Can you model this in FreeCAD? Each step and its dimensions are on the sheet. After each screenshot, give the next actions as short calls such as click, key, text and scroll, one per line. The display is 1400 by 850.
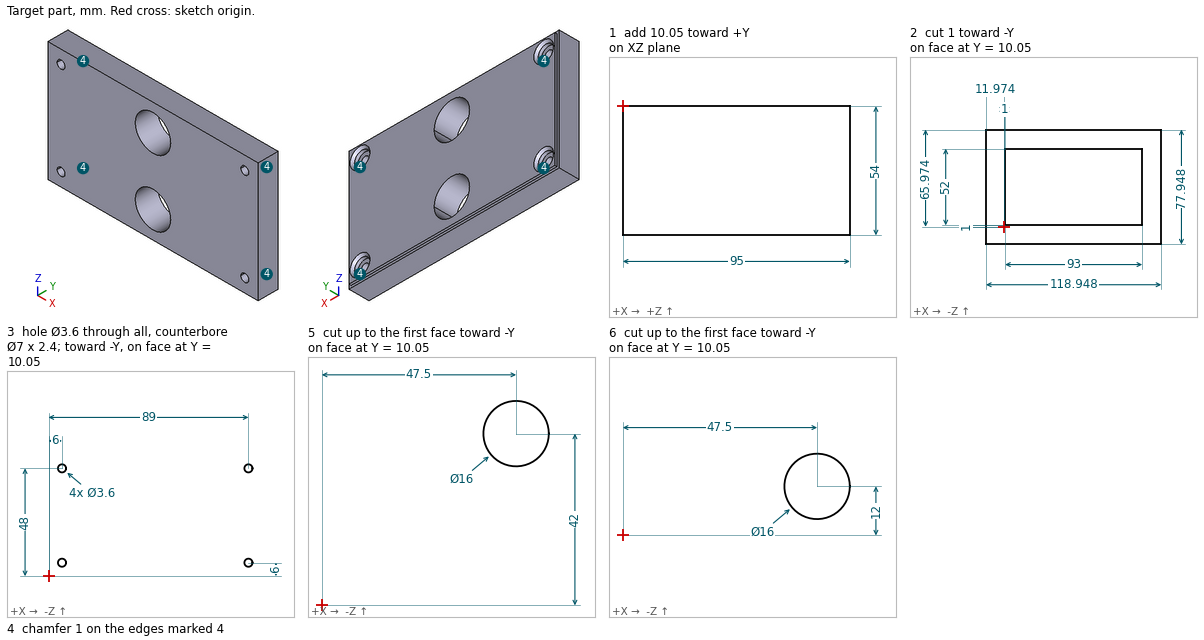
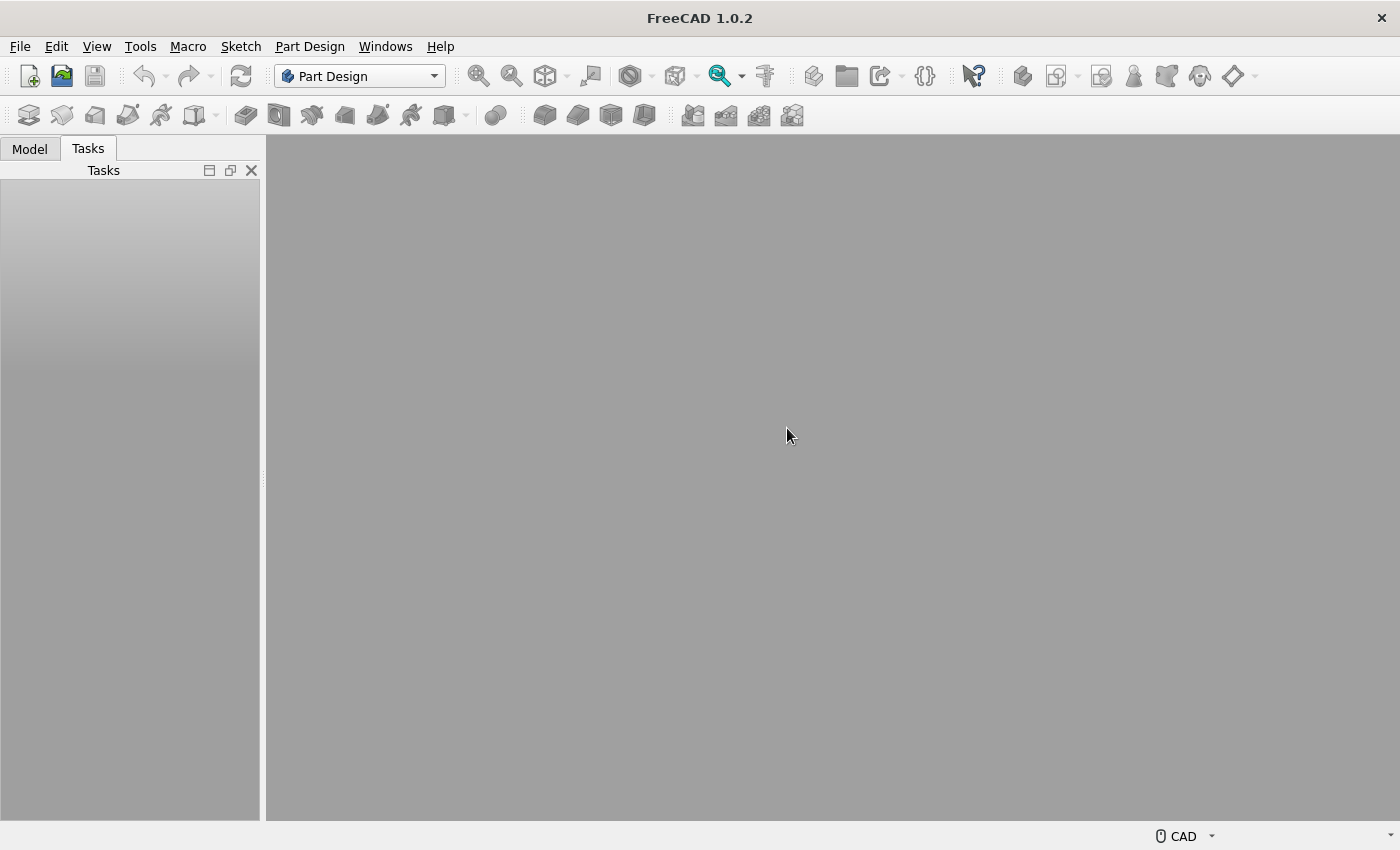
click(29, 76)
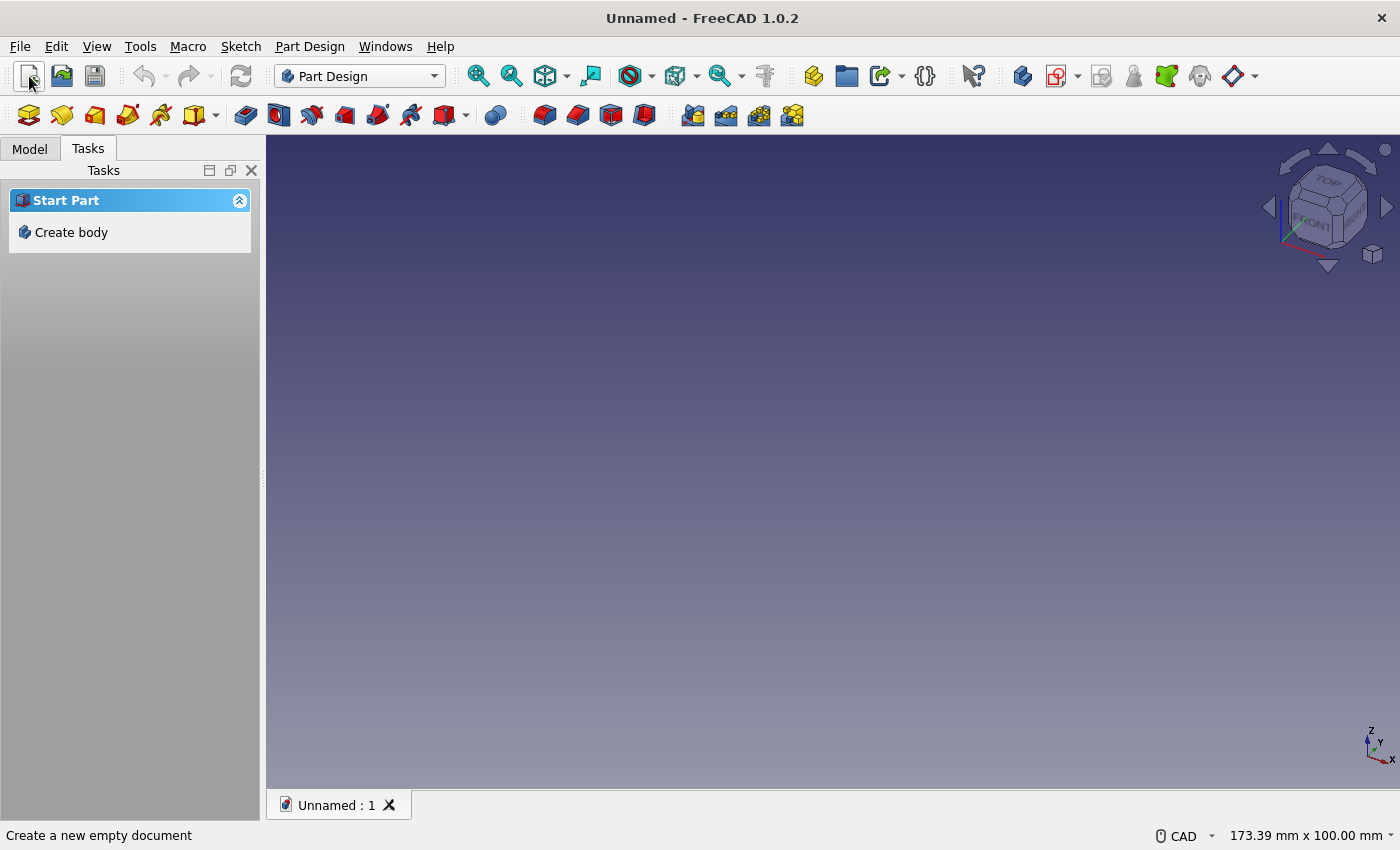
click(1056, 76)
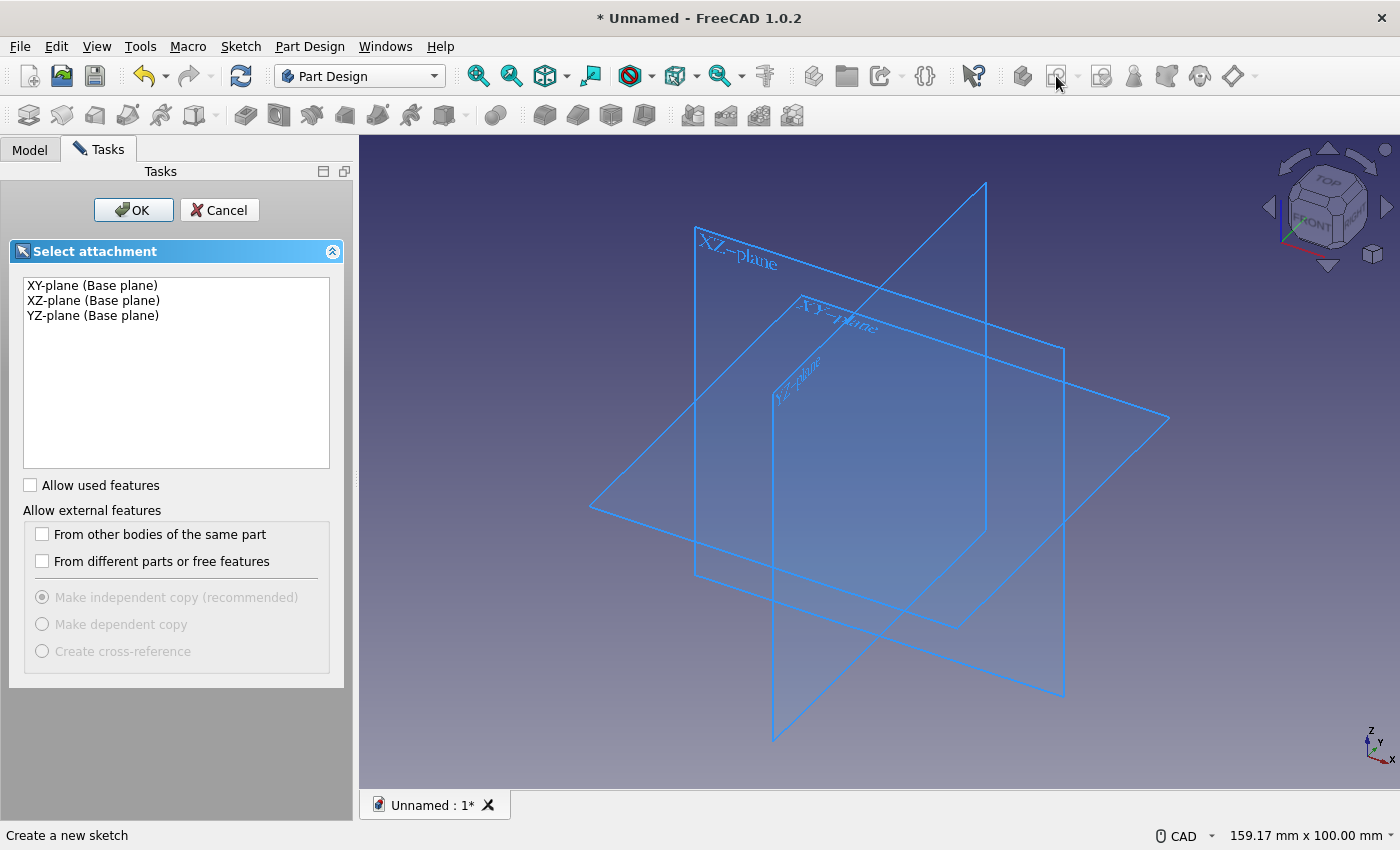
click(84, 300)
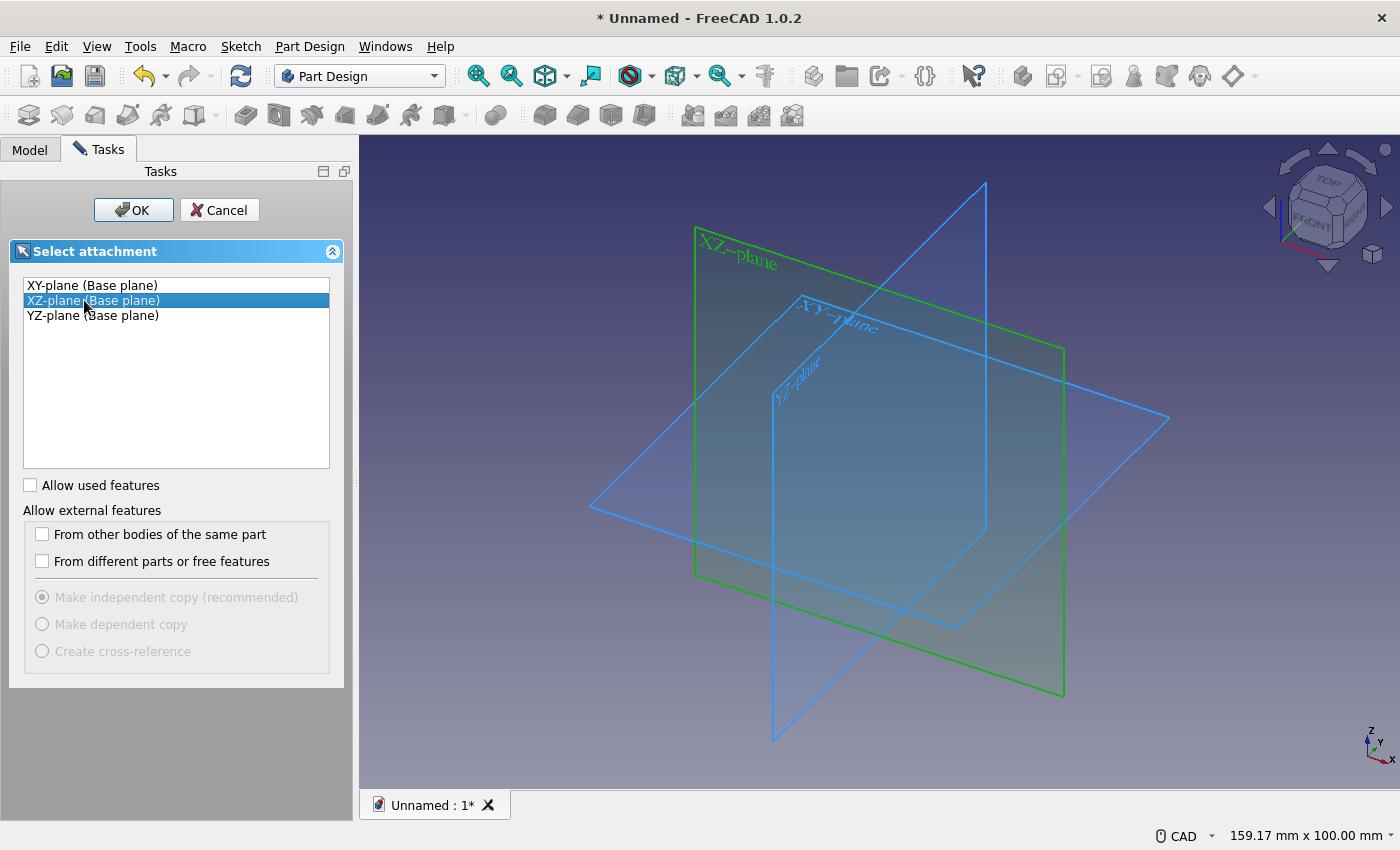
click(134, 210)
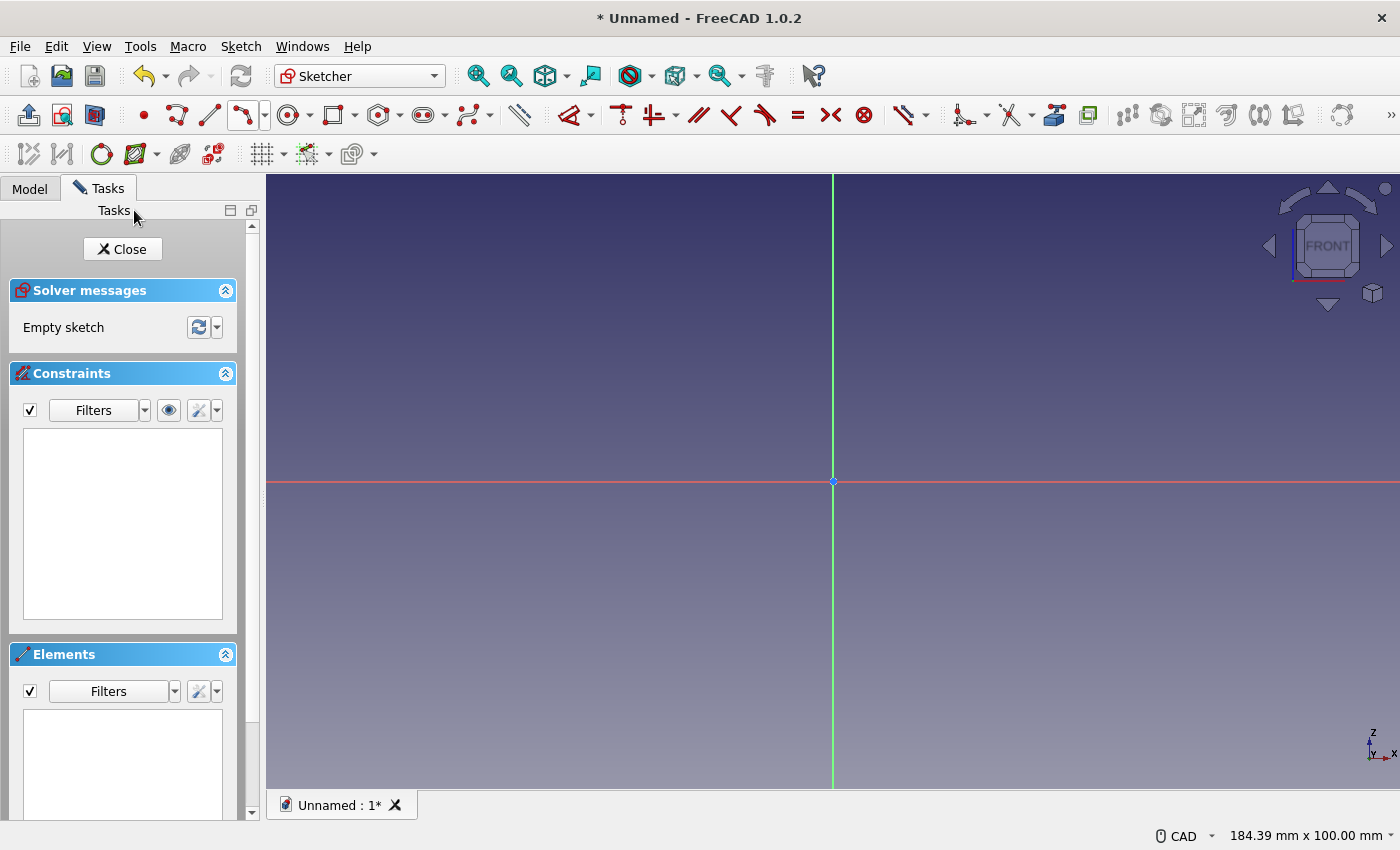
scroll(294, 202, down, 2)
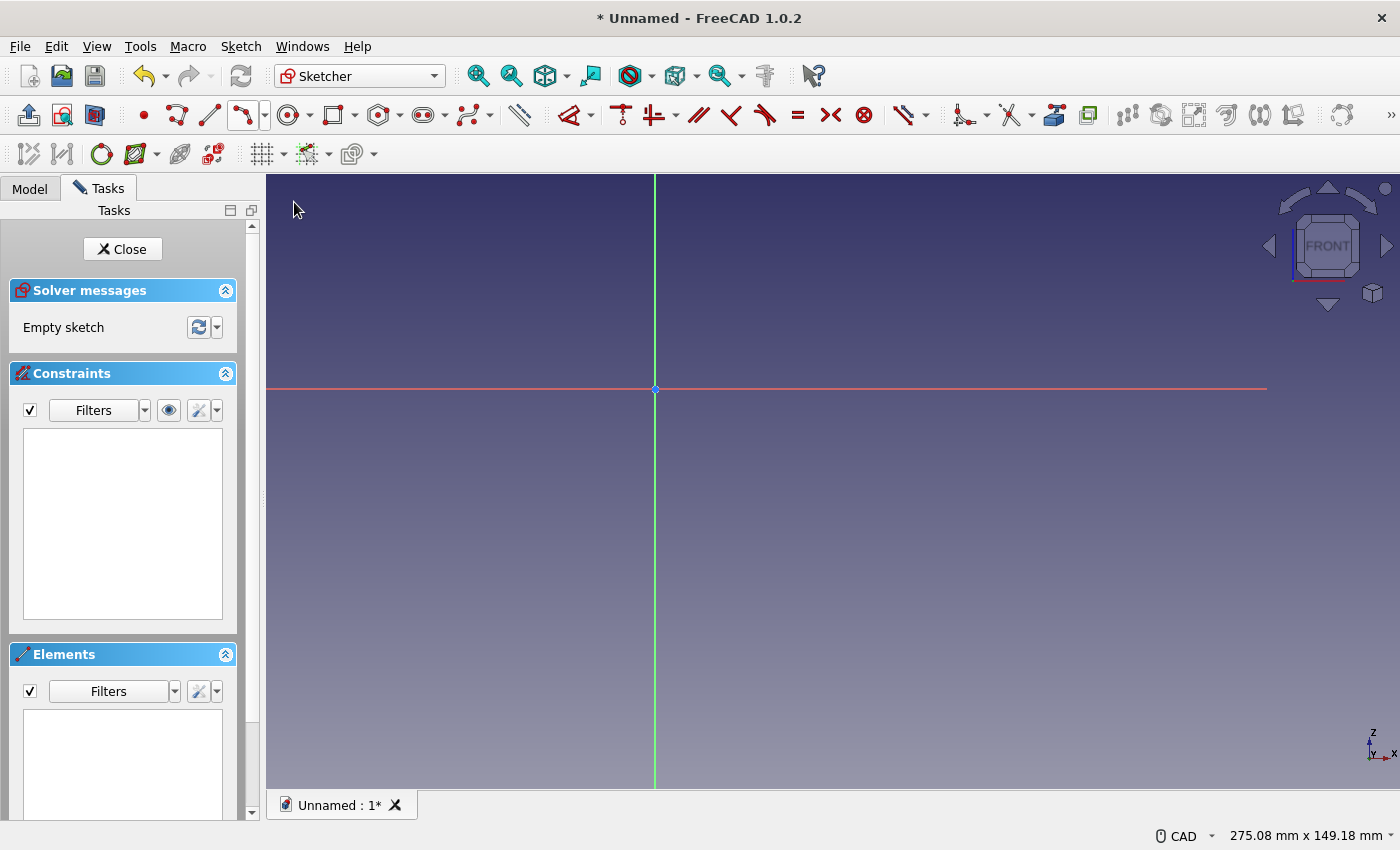
scroll(956, 524, up, 3)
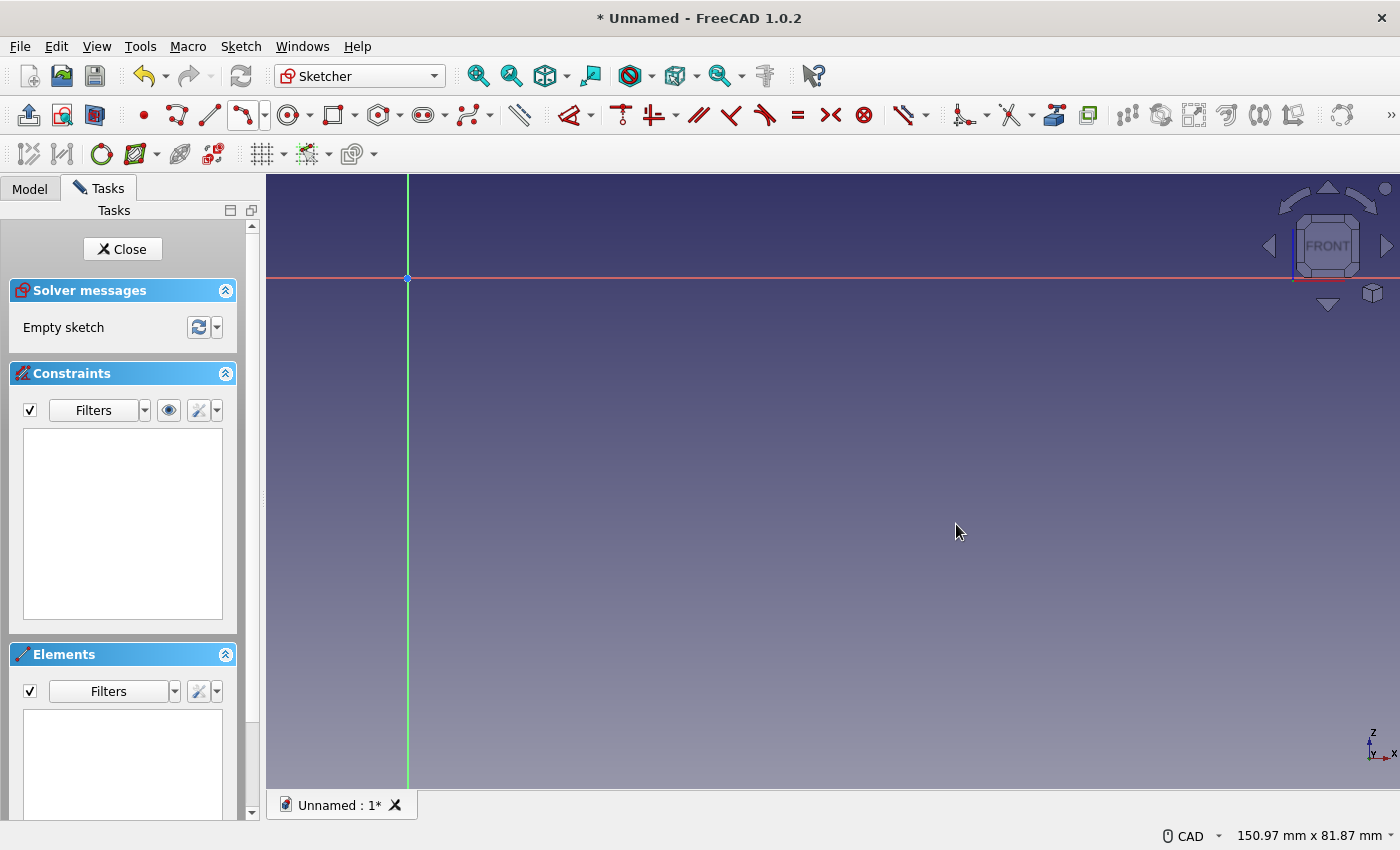
click(332, 116)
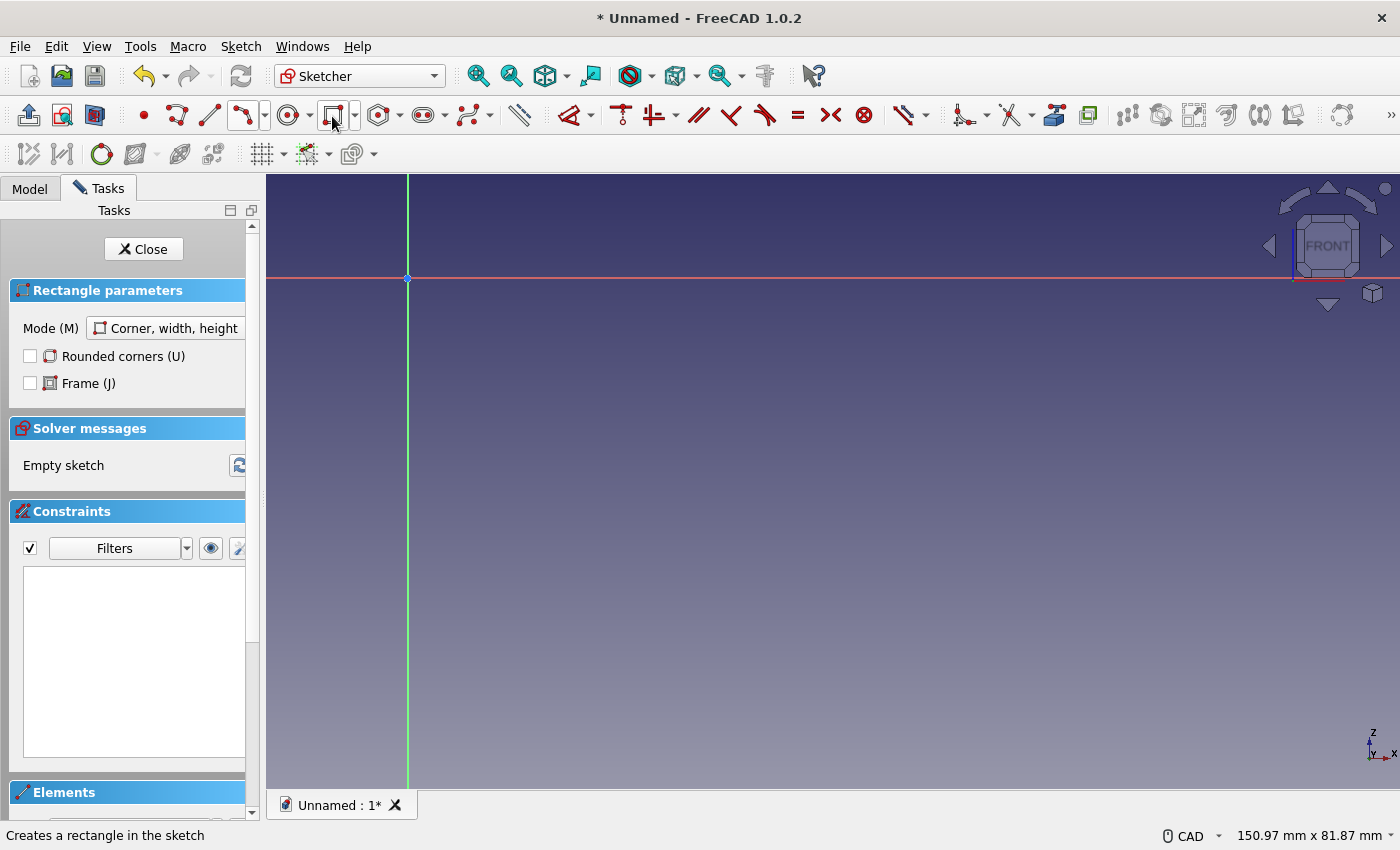
click(408, 278)
move(1121, 684)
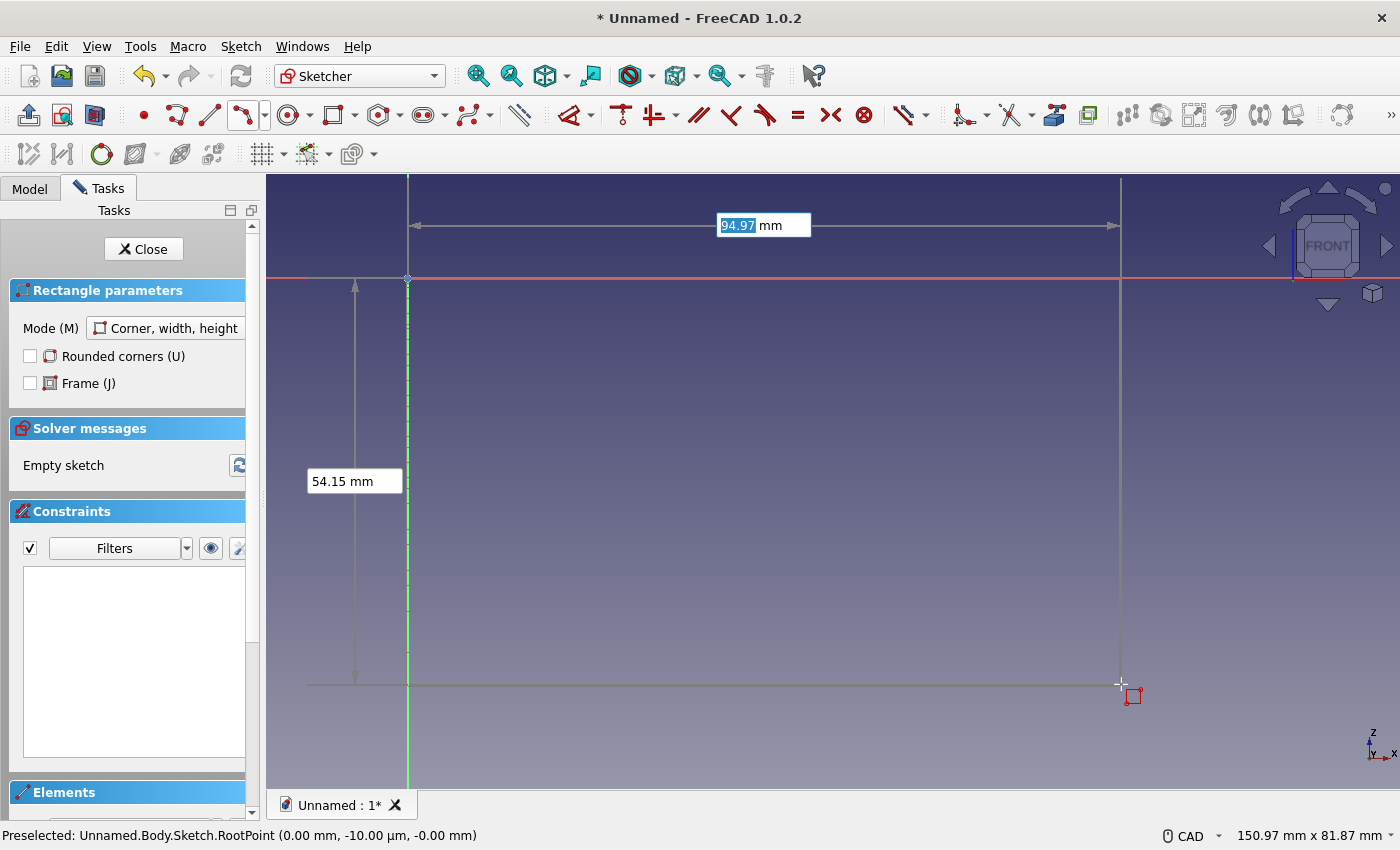
text(95)
key(Tab)
text(54)
key(Return)
key(Escape)